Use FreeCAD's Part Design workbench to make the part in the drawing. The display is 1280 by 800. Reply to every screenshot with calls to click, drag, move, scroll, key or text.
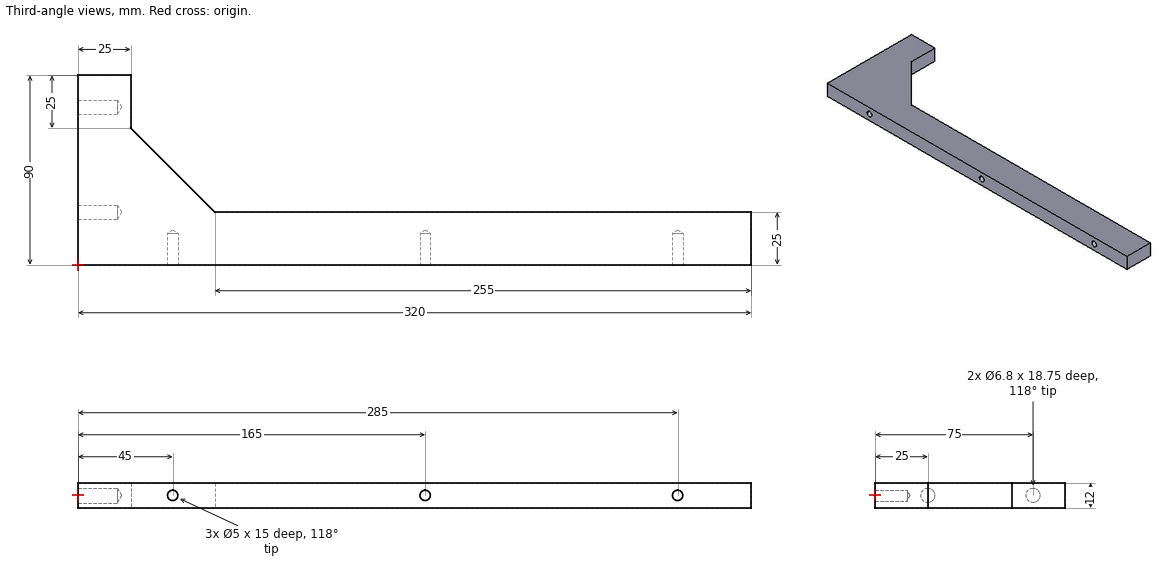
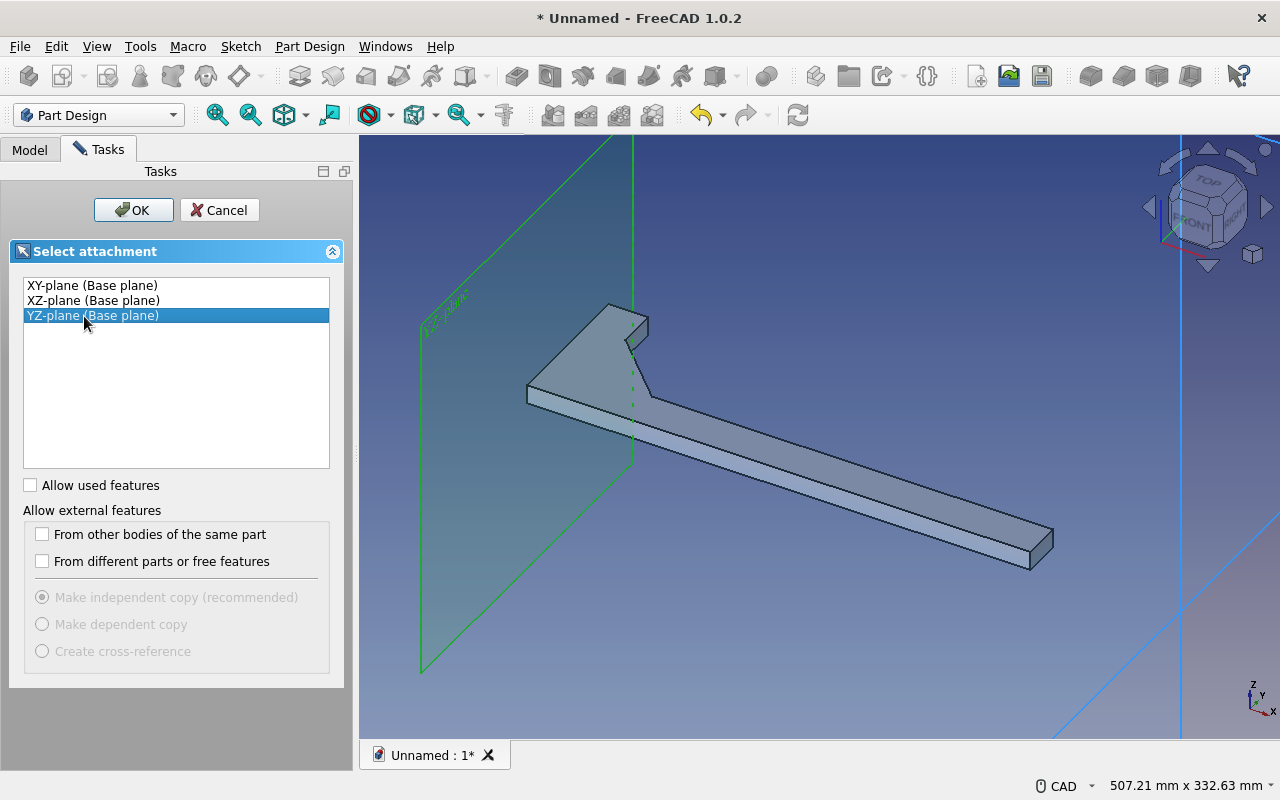
click(134, 210)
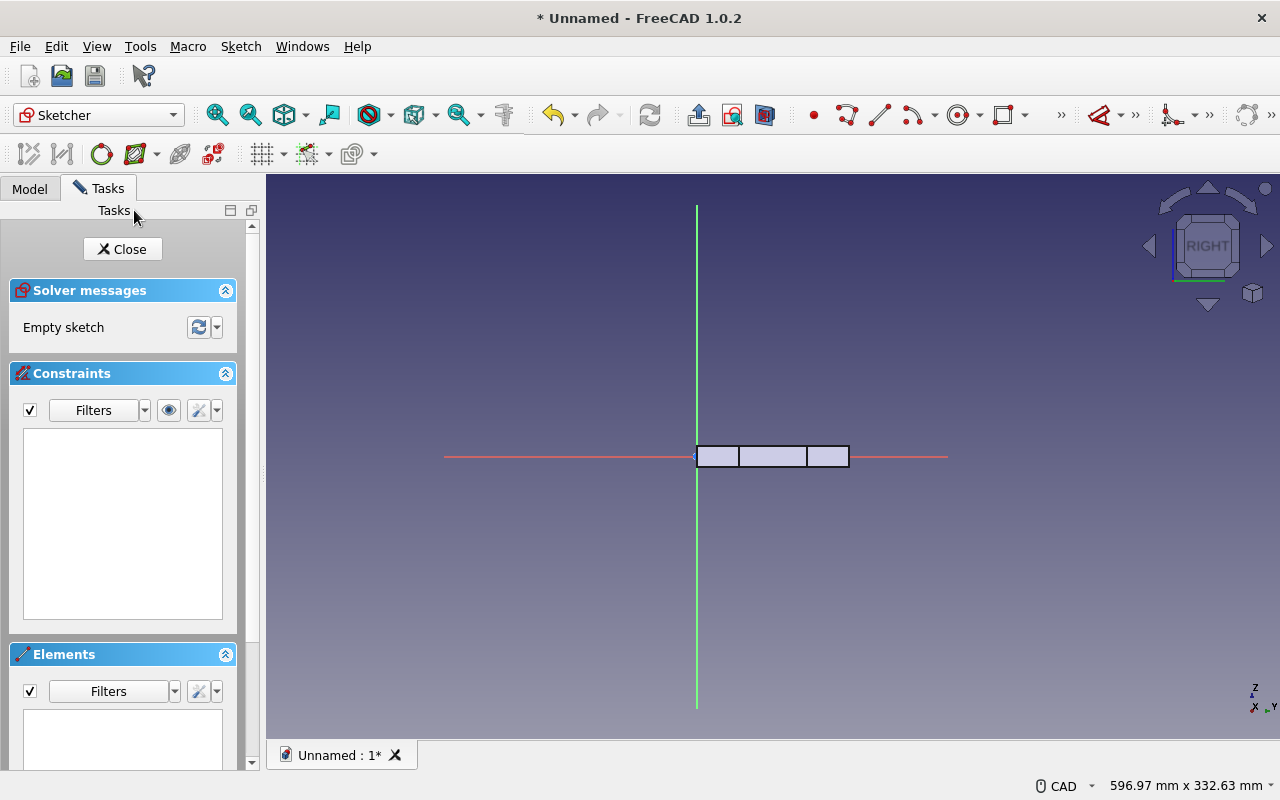
key(q)
key(s)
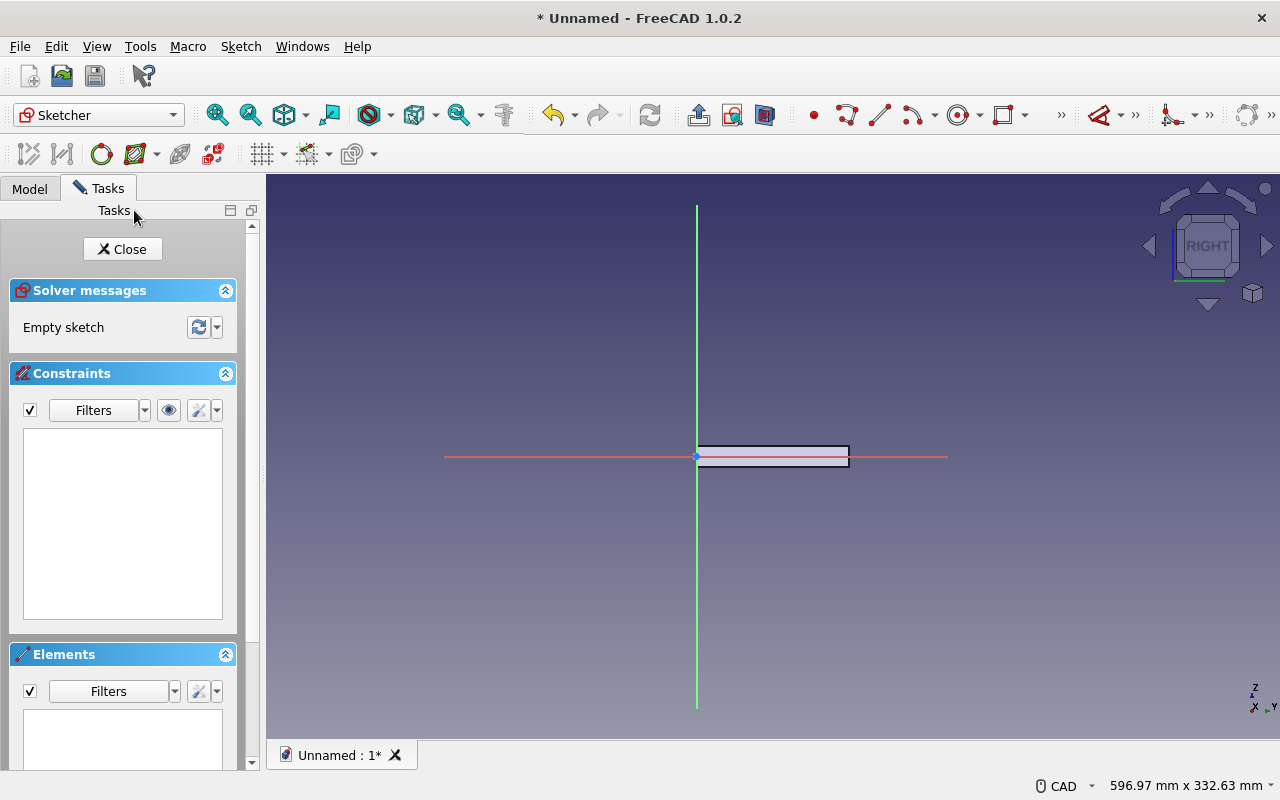
scroll(782, 456, up, 7)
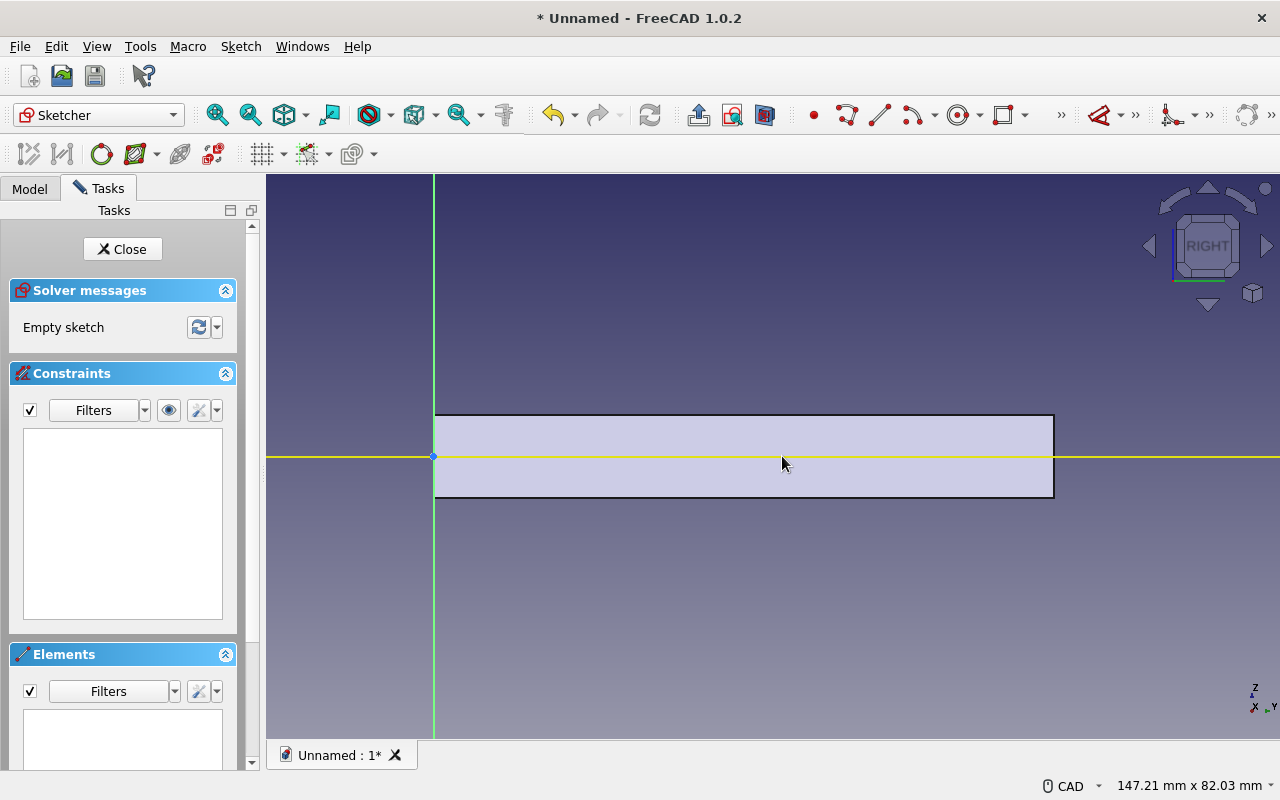
click(958, 116)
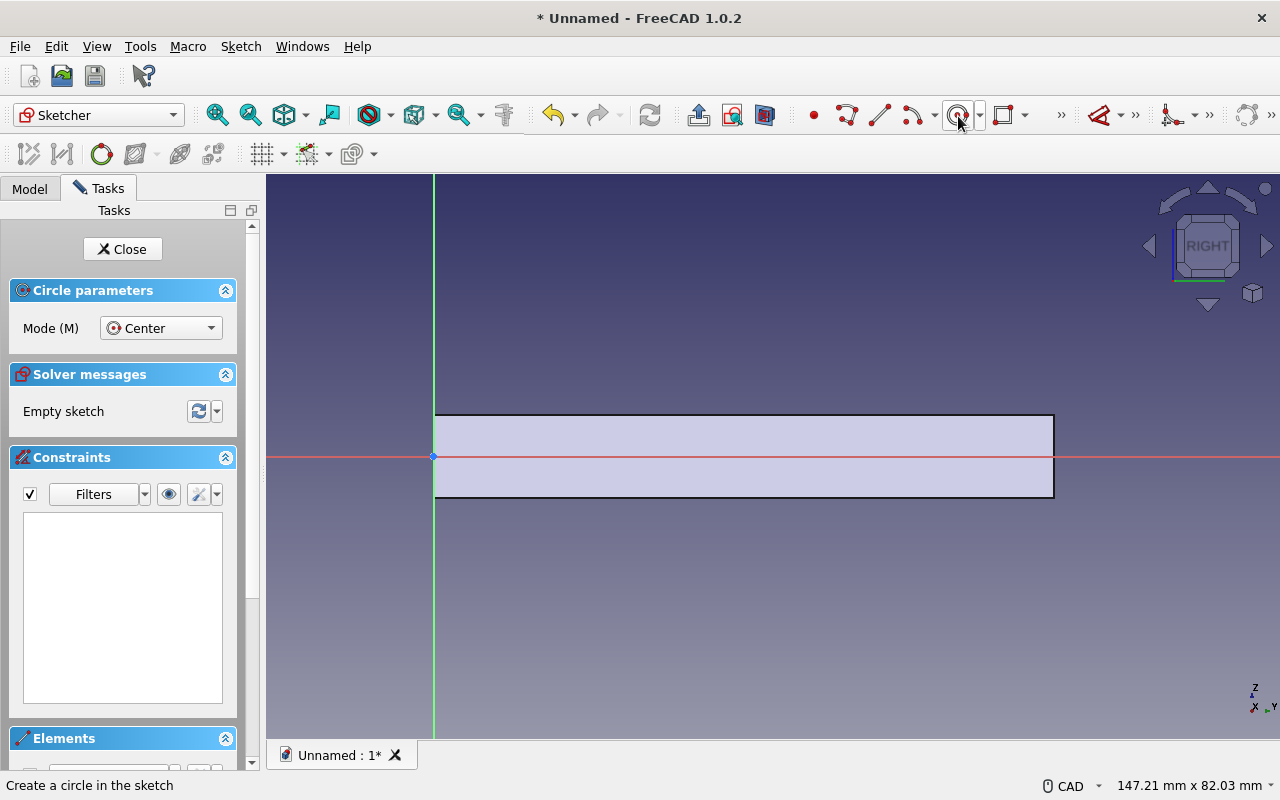
click(951, 456)
click(967, 440)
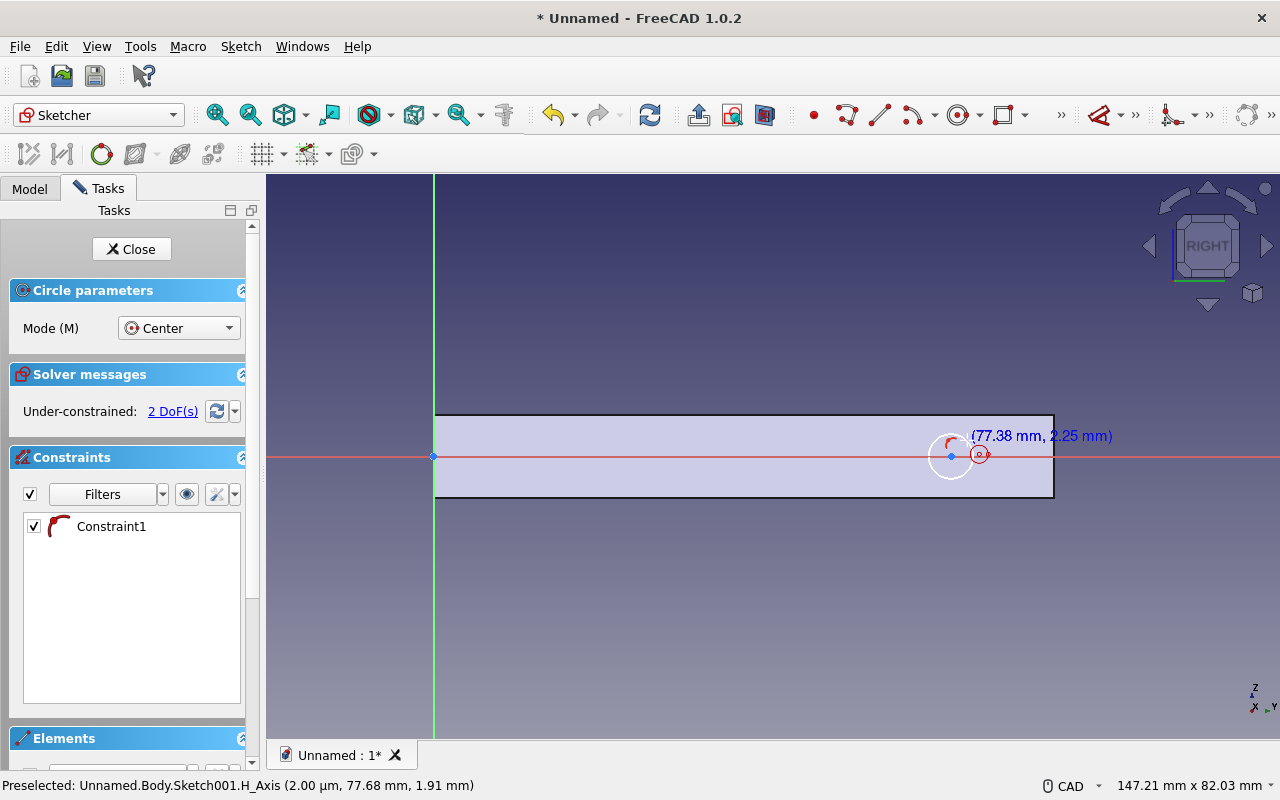
click(606, 456)
click(623, 440)
key(Escape)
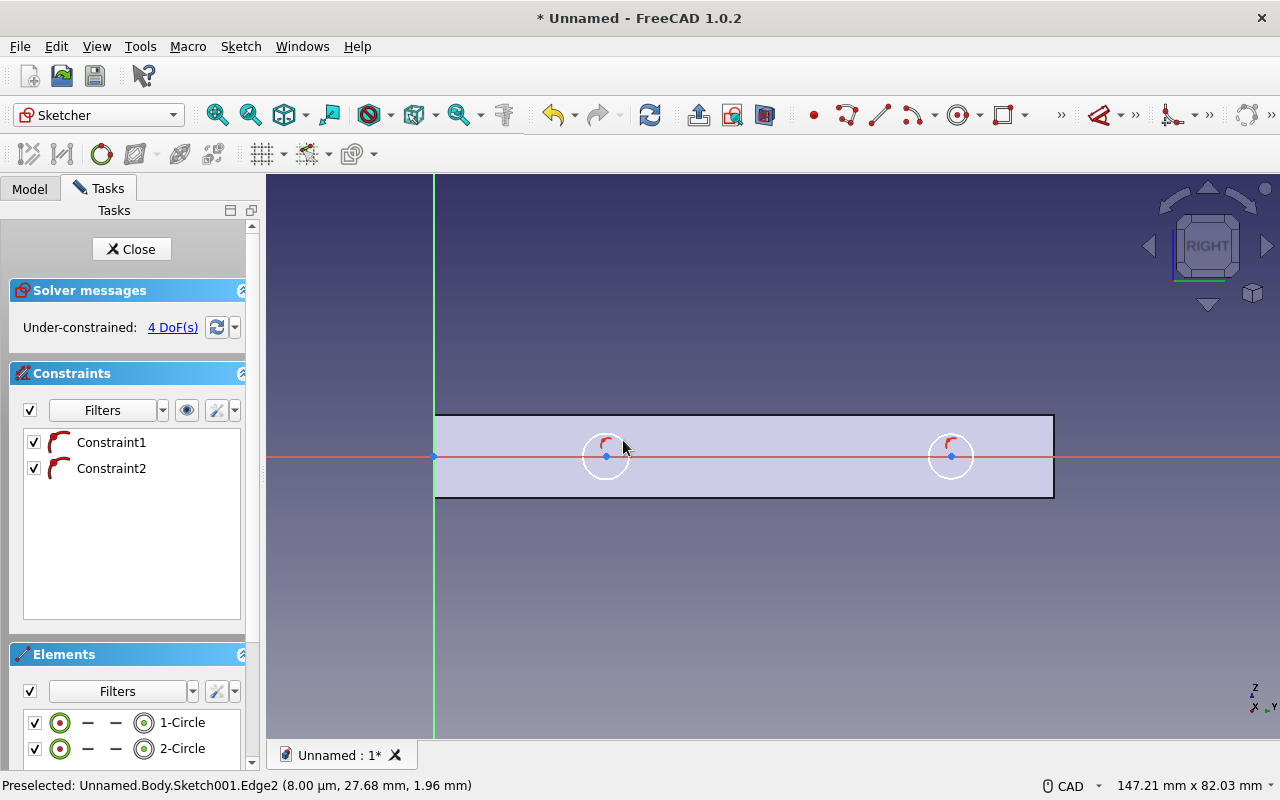
click(967, 441)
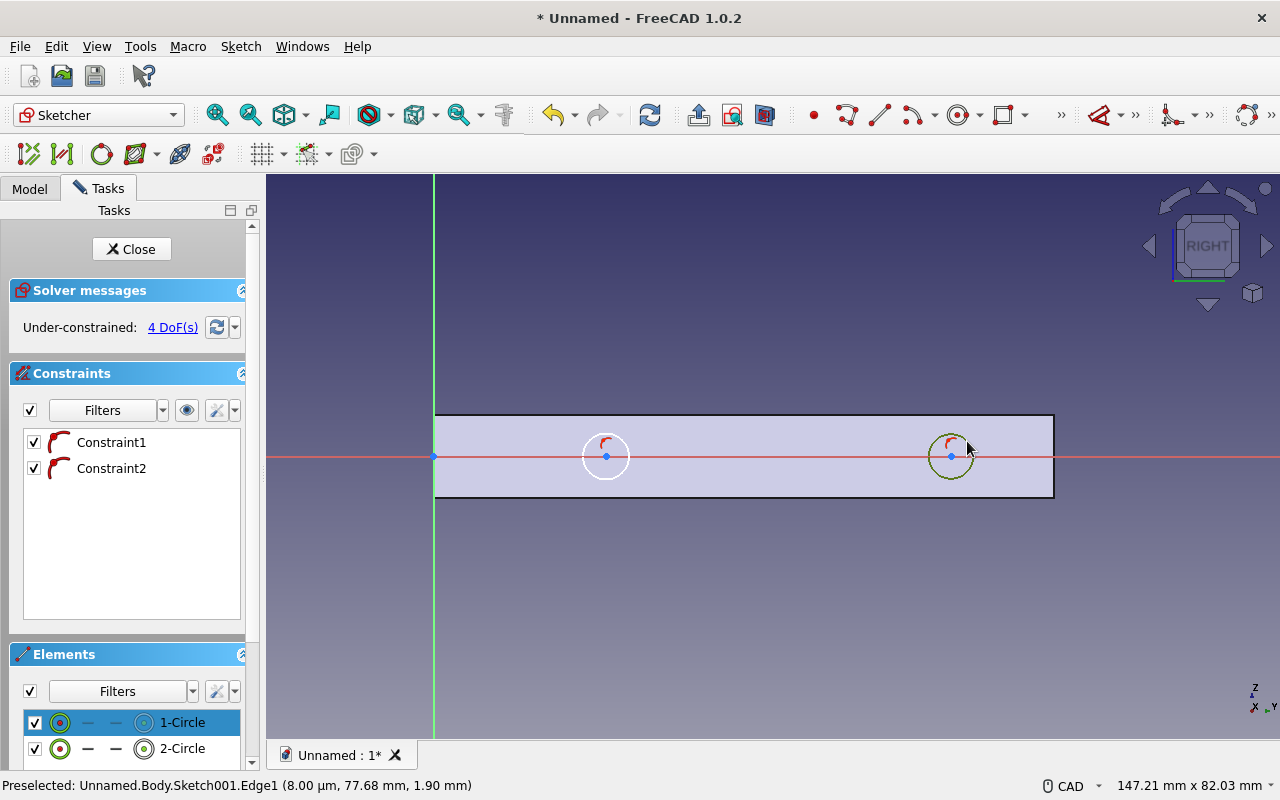
click(622, 440)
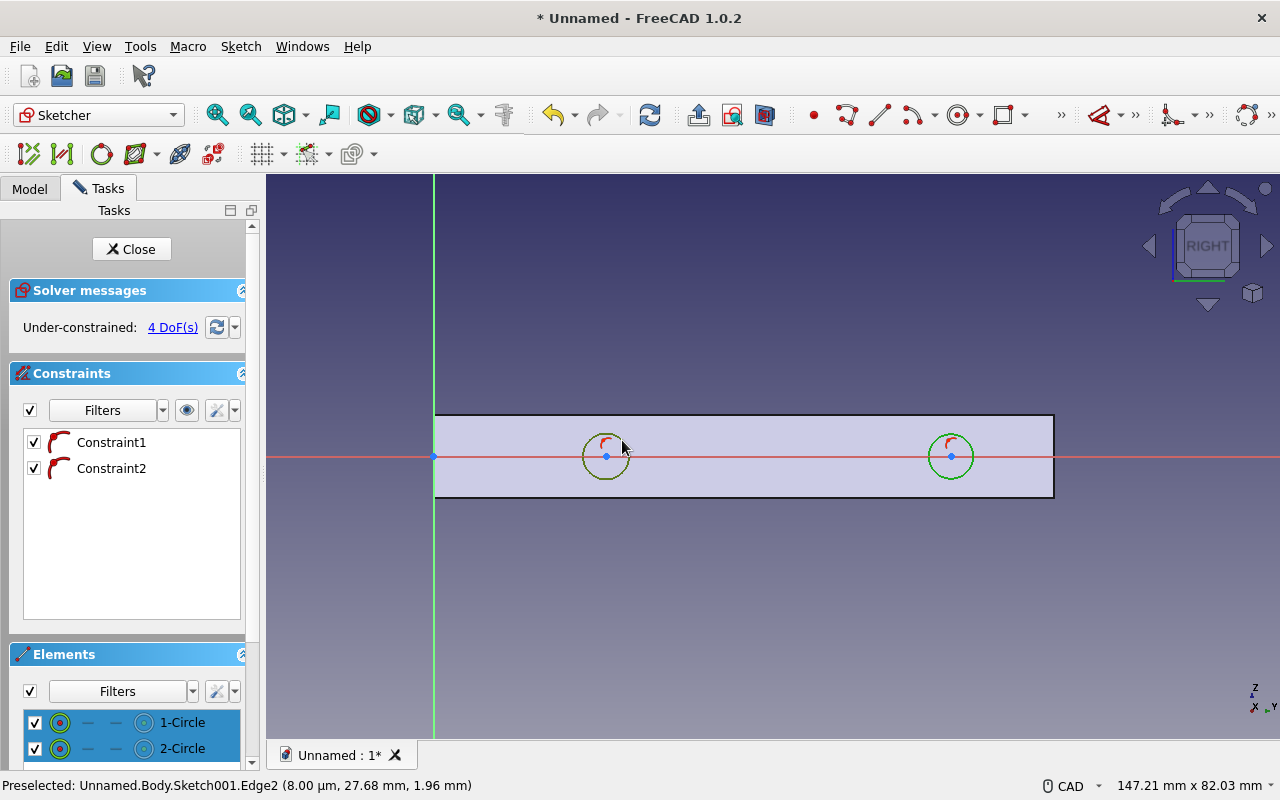
key(e)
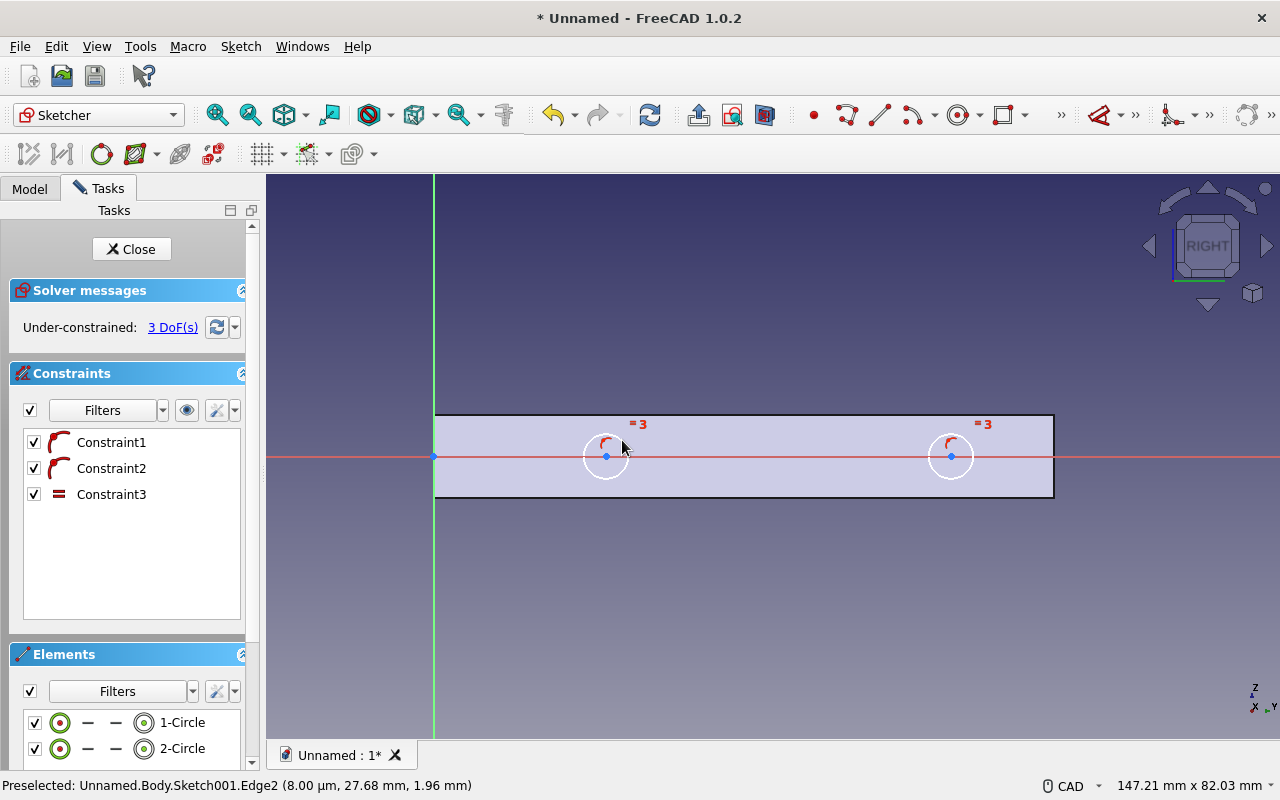
click(1098, 116)